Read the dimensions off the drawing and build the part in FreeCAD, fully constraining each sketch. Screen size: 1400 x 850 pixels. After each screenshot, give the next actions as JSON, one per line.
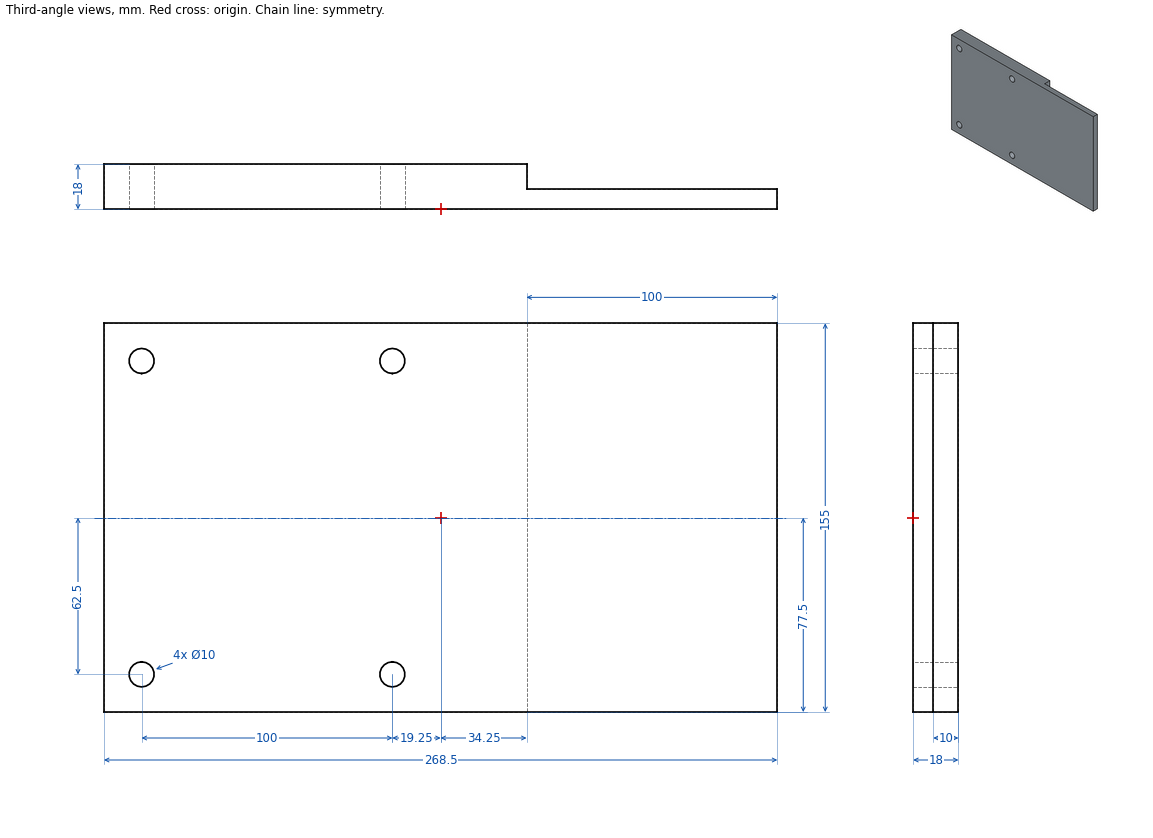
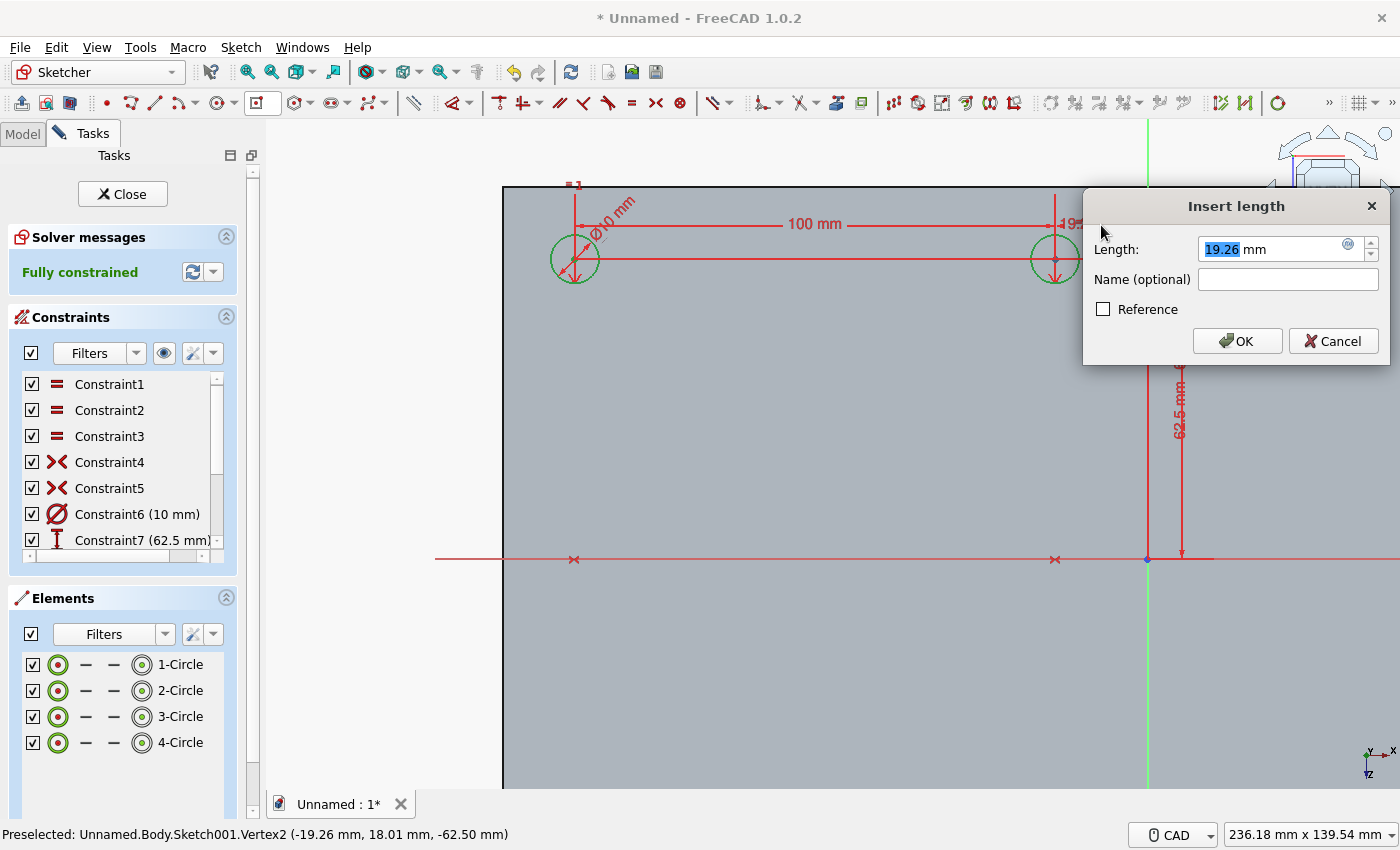
{"action": "type", "text": "19.25"}
{"action": "key", "text": "Return"}
{"action": "key", "text": "Escape"}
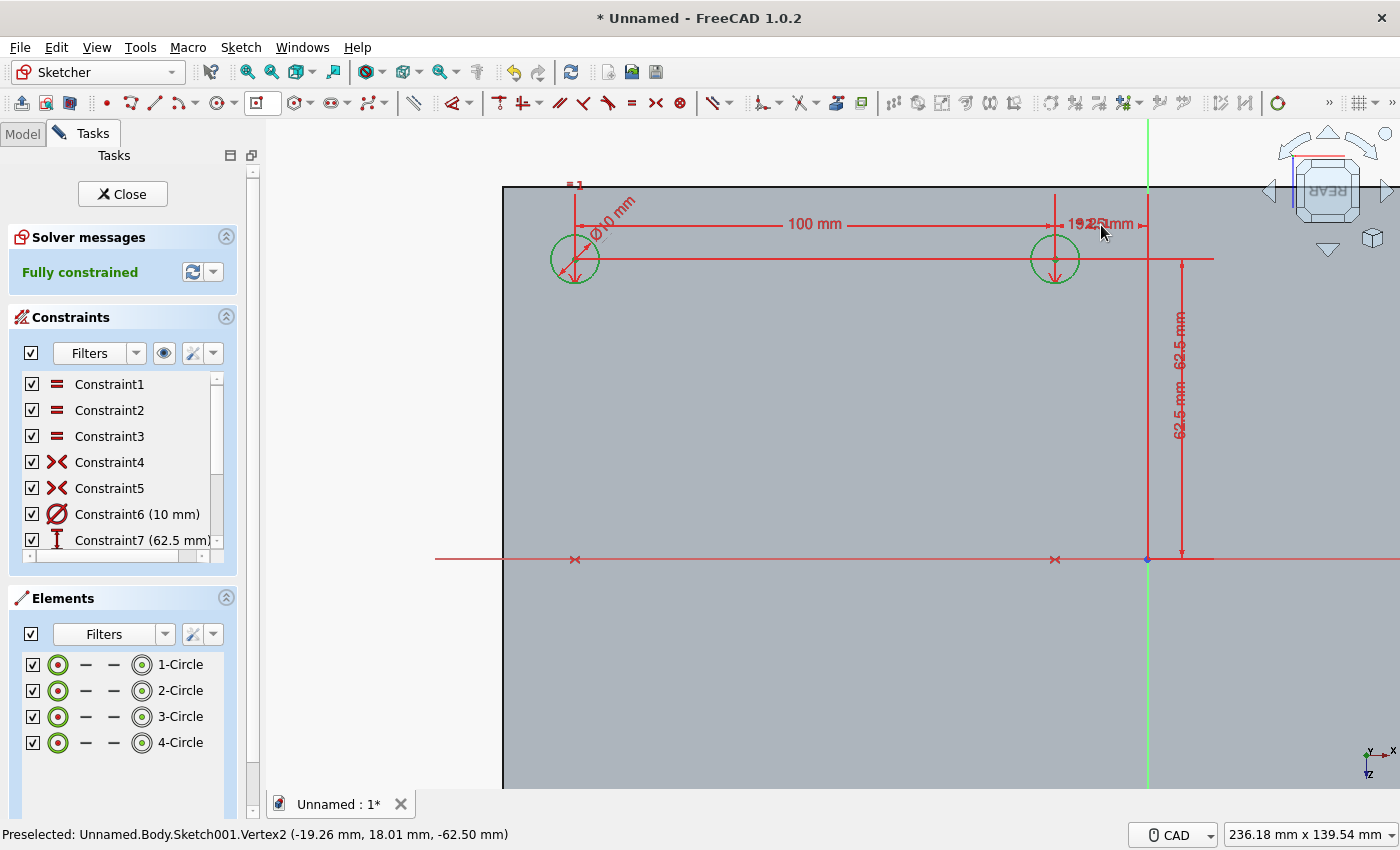
{"action": "left_click", "coordinate": [123, 194]}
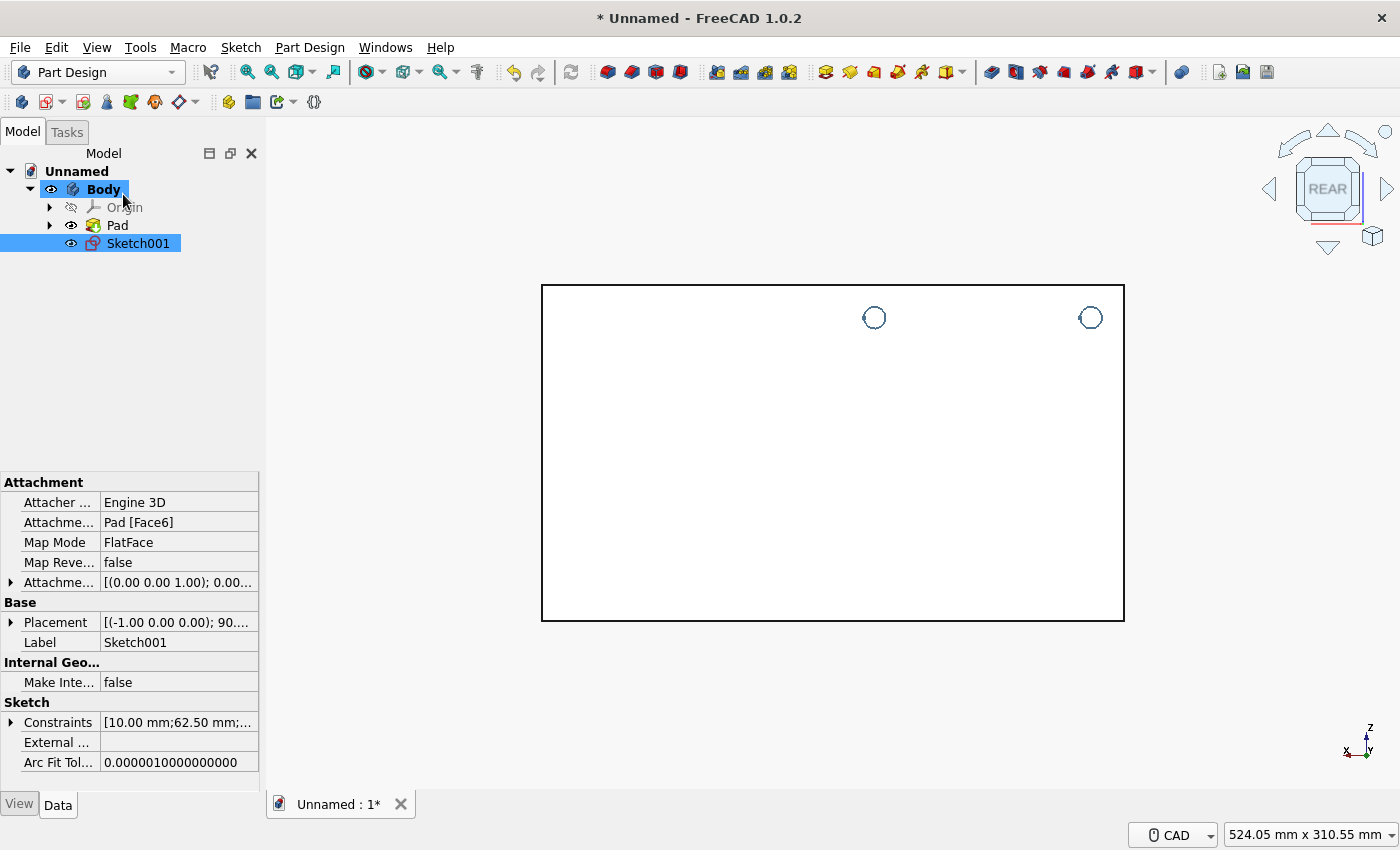
{"action": "left_click", "coordinate": [992, 72]}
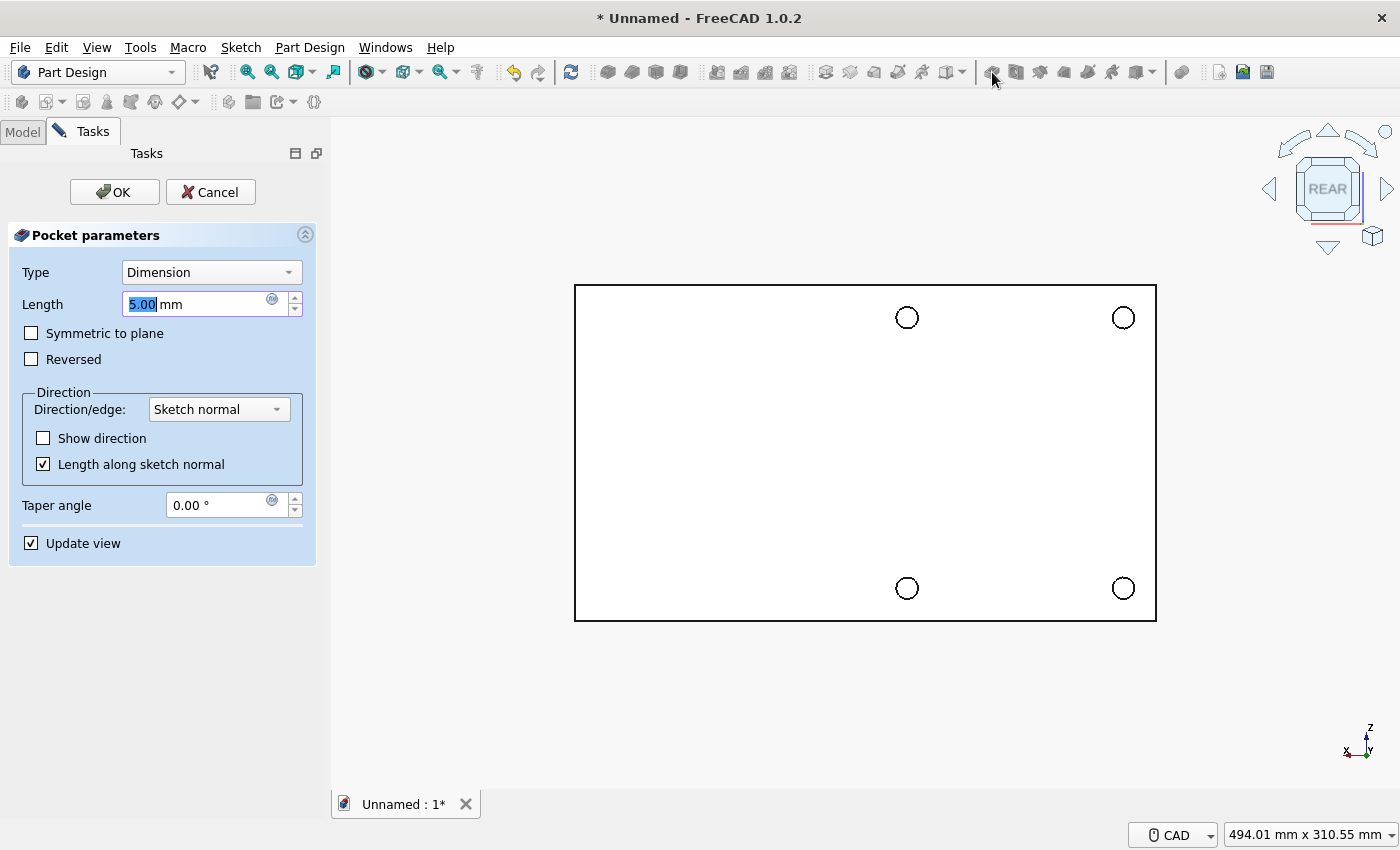
{"action": "type", "text": "18"}
{"action": "key", "text": "Tab"}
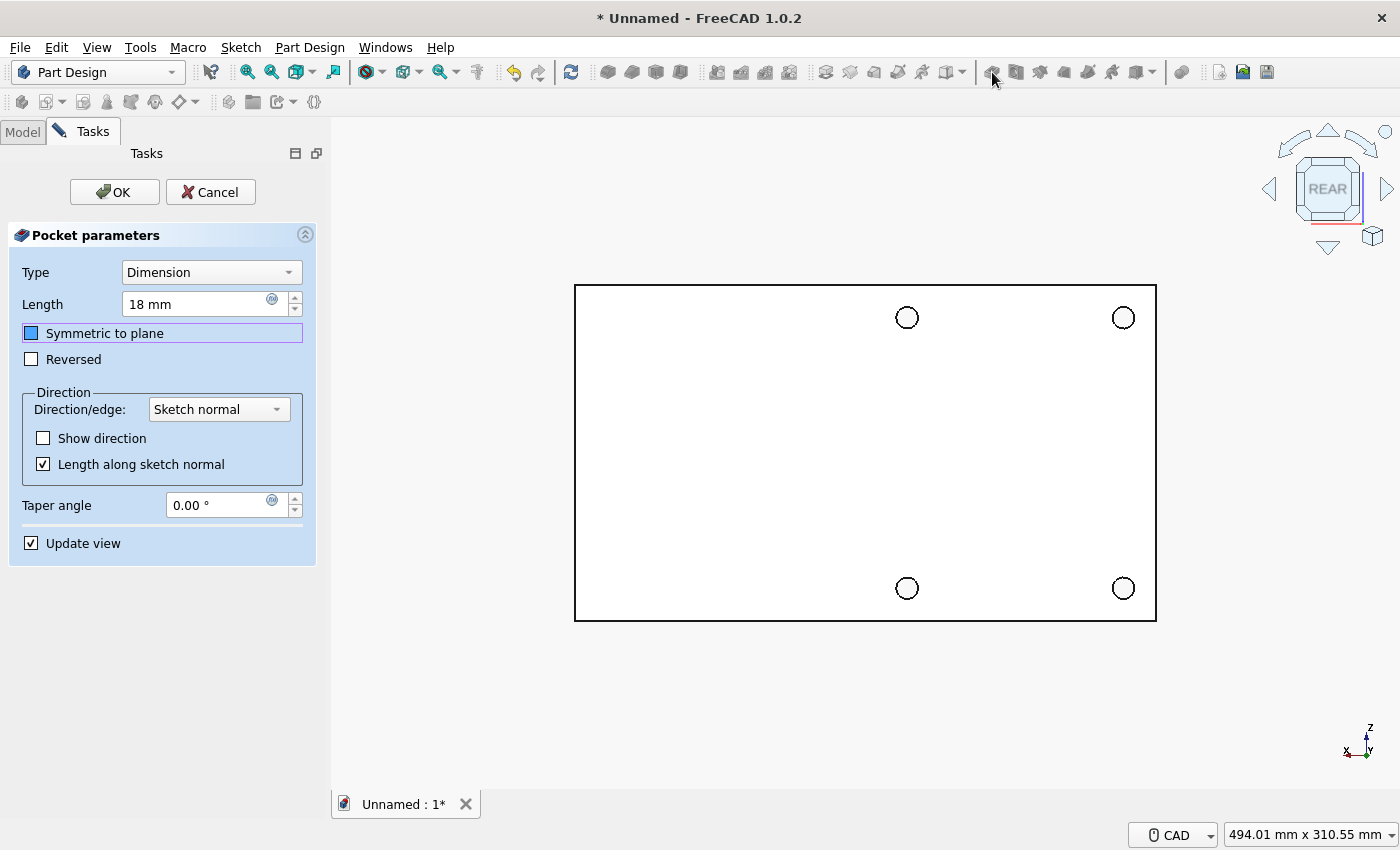
{"action": "left_click", "coordinate": [115, 192]}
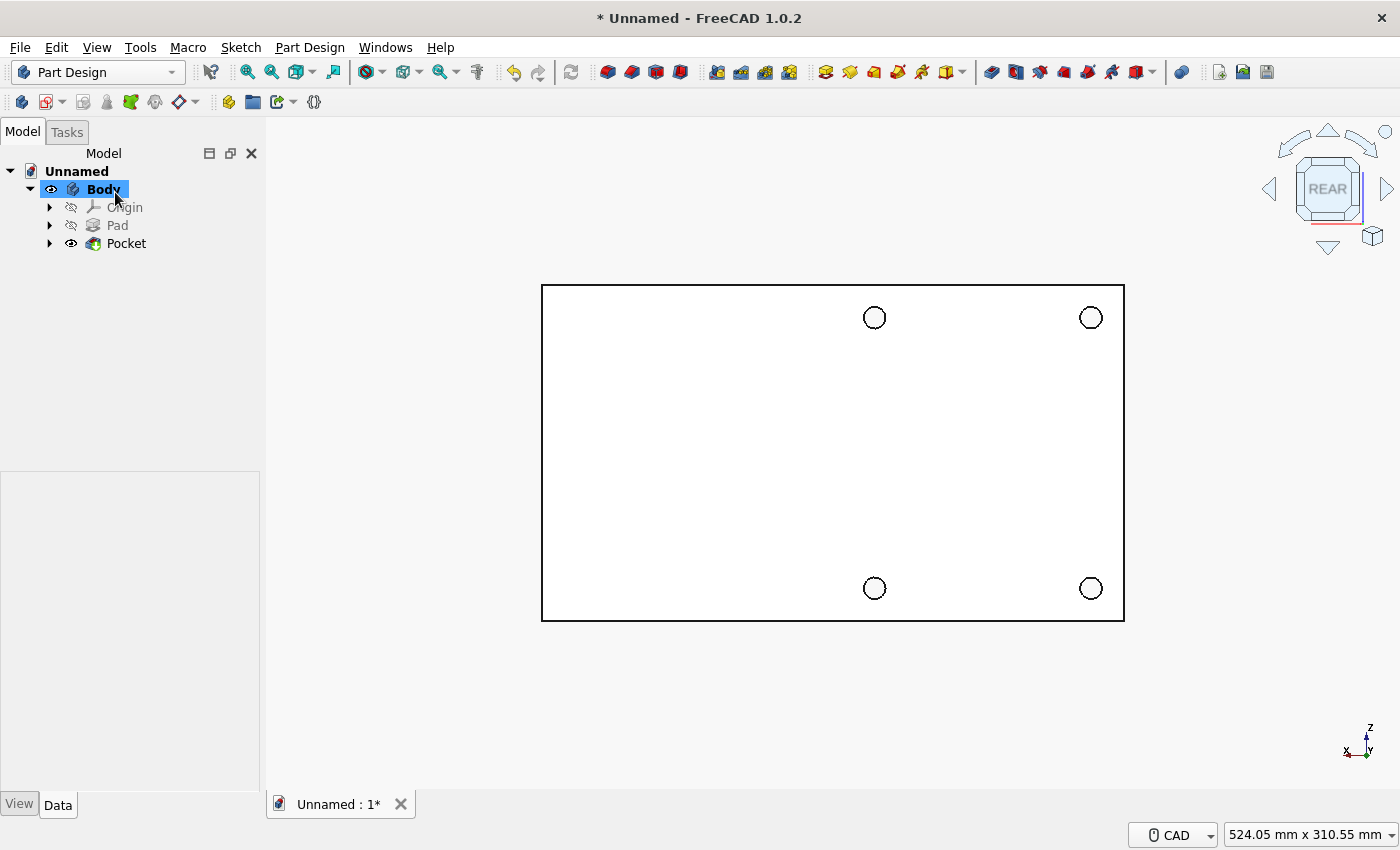
{"action": "left_click", "coordinate": [750, 452]}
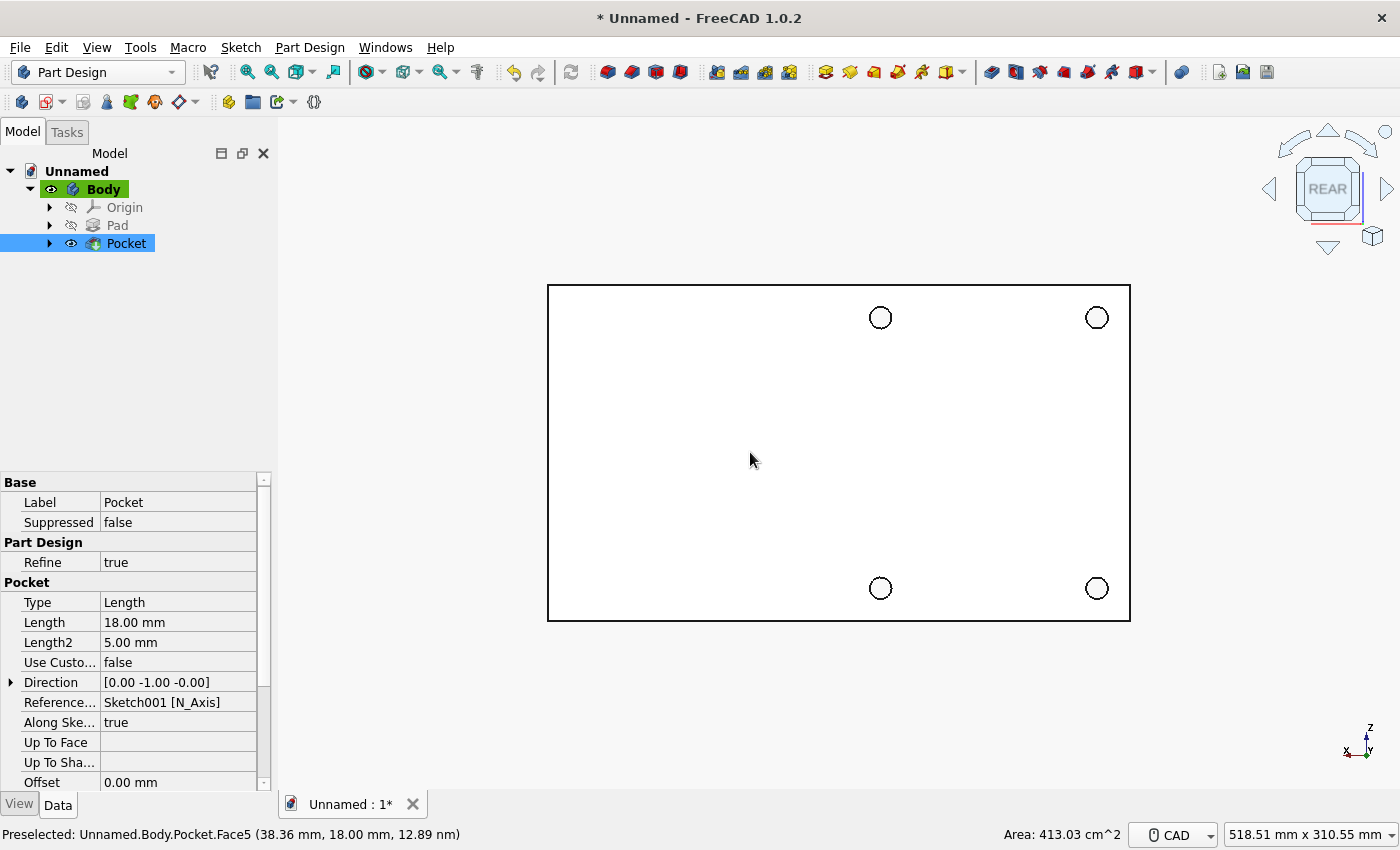
{"action": "left_click", "coordinate": [46, 102]}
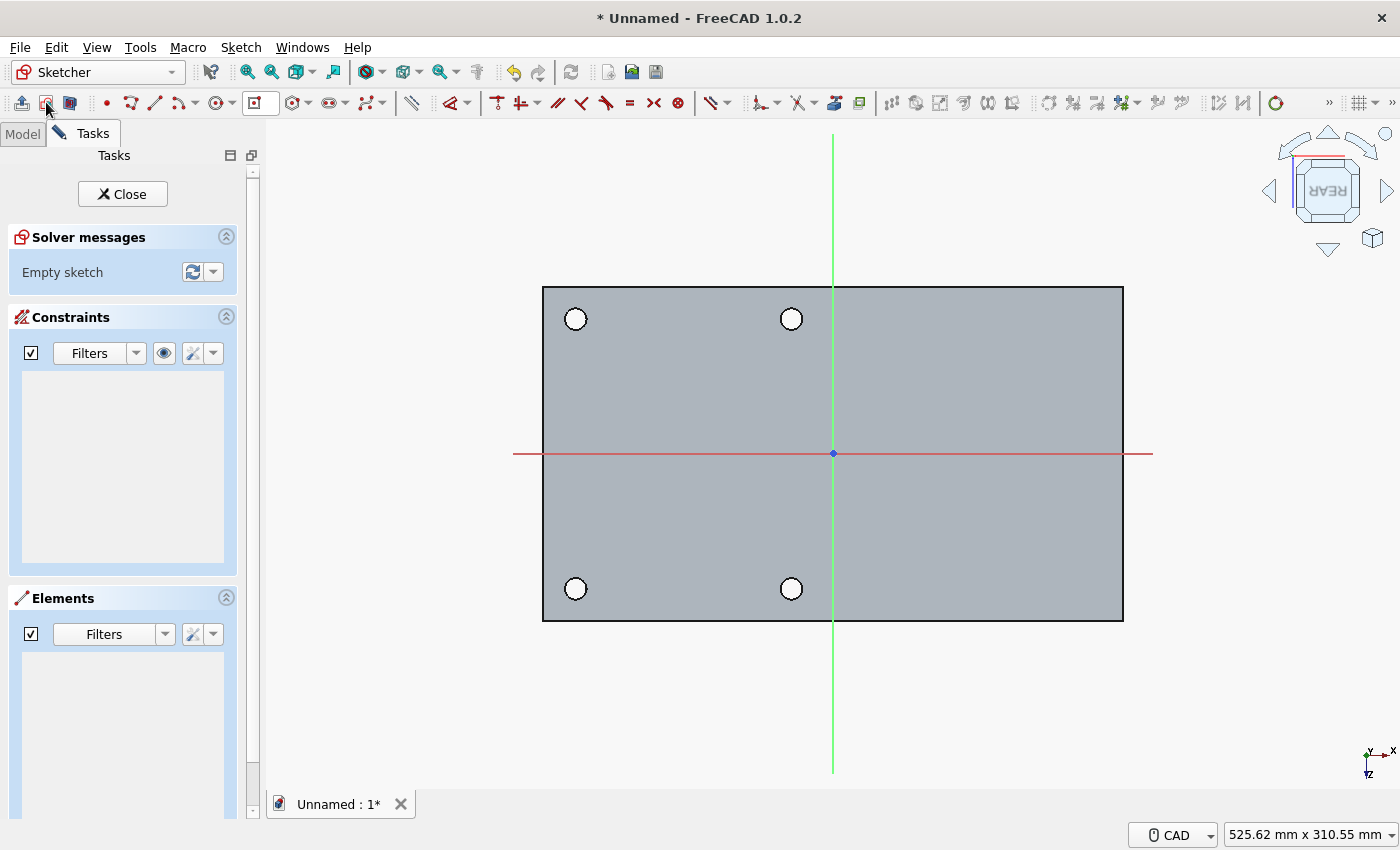
{"action": "key", "text": "g r"}